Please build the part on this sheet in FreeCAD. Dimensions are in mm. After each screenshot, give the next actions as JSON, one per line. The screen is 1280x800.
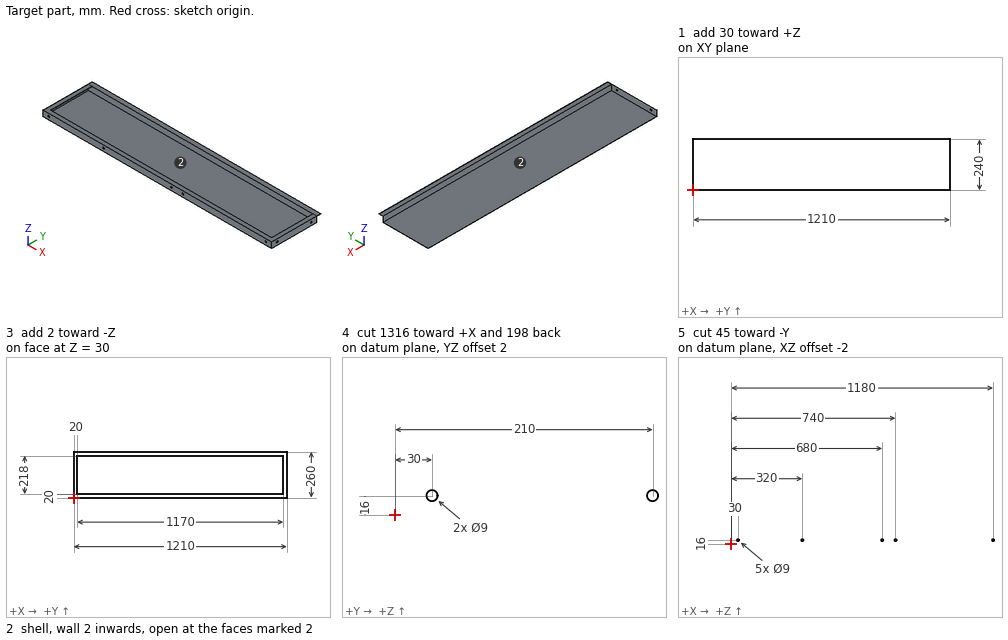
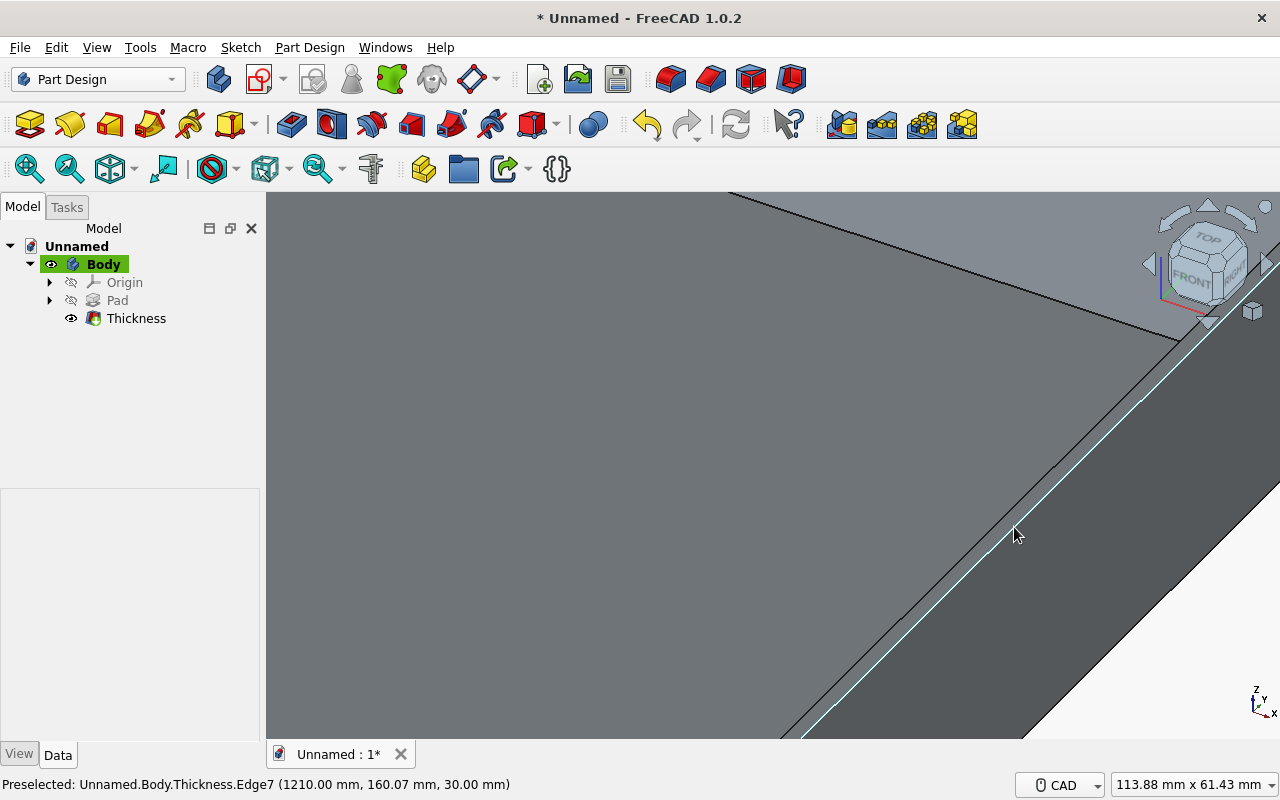
{"action": "scroll", "coordinate": [994, 539], "scroll_direction": "up", "scroll_amount": 4}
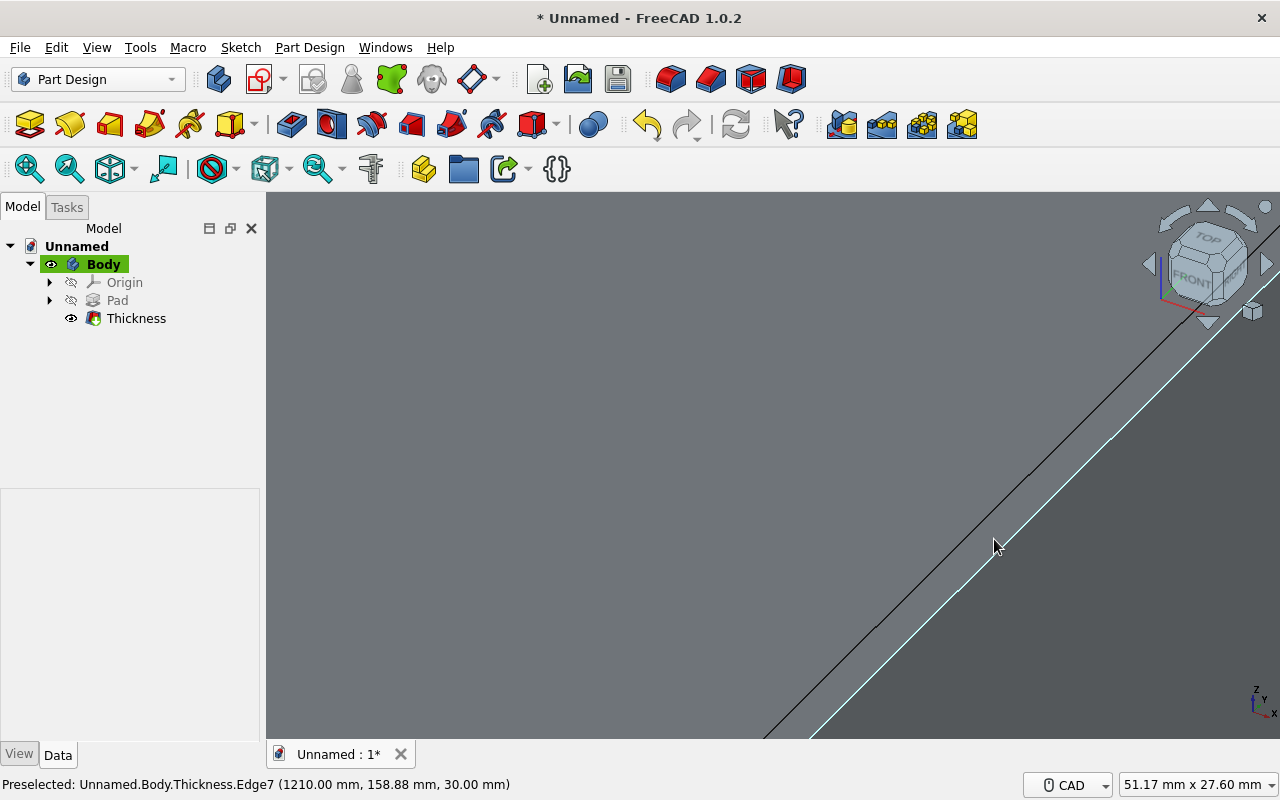
{"action": "left_click", "coordinate": [994, 539]}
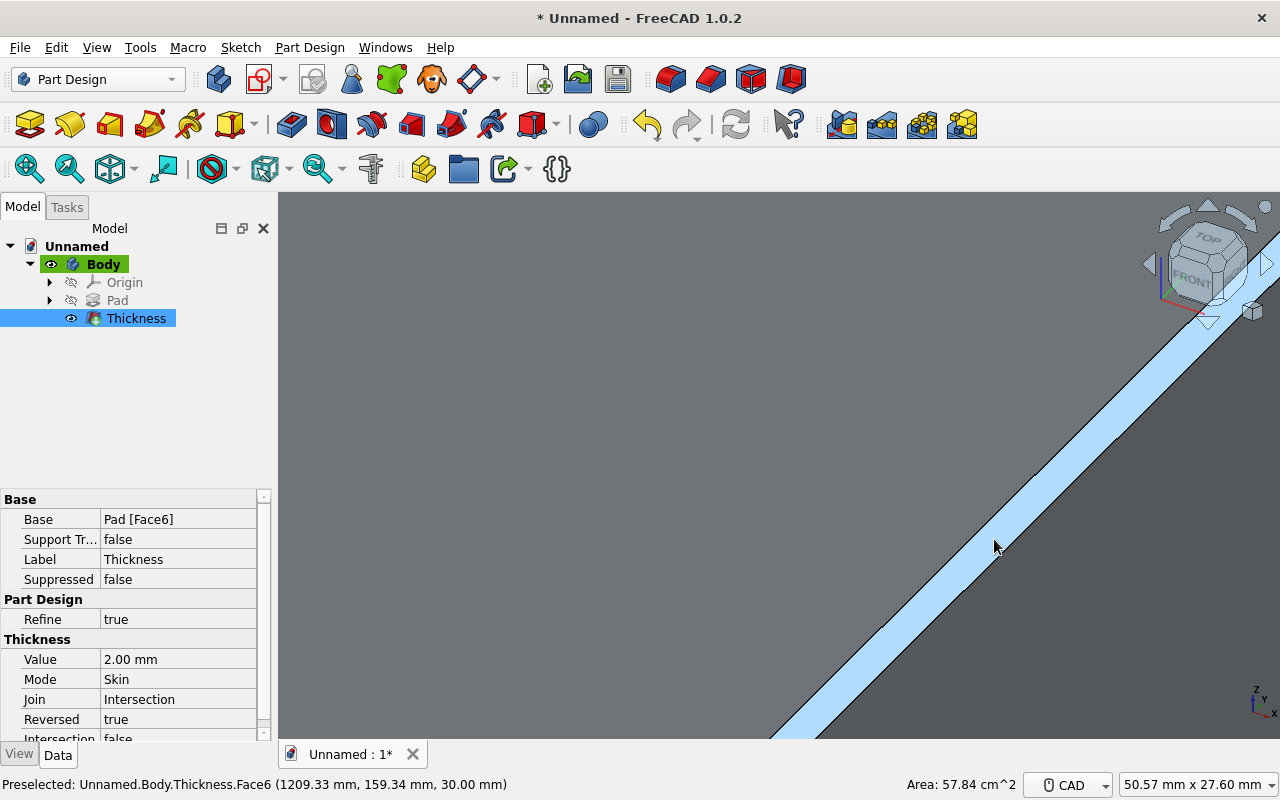
{"action": "left_click", "coordinate": [260, 80]}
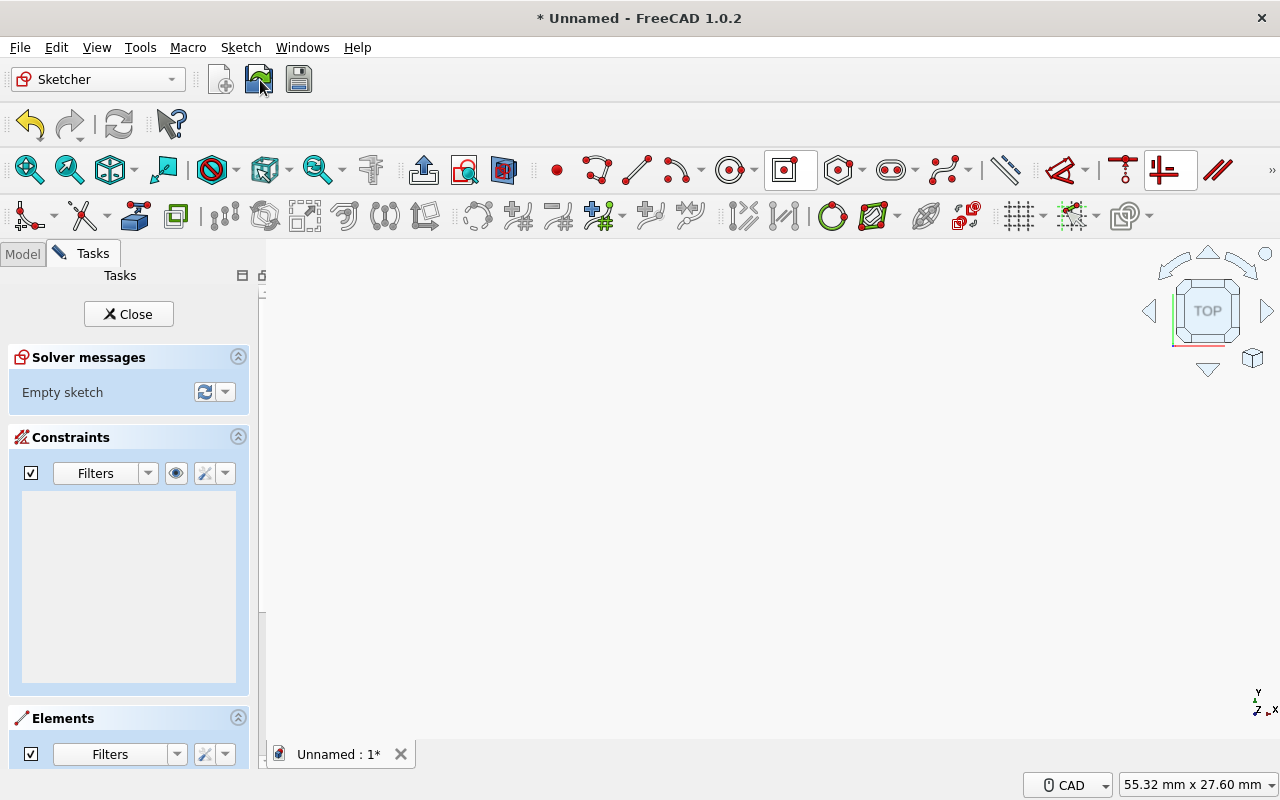
{"action": "scroll", "coordinate": [1015, 372], "scroll_direction": "down", "scroll_amount": 17}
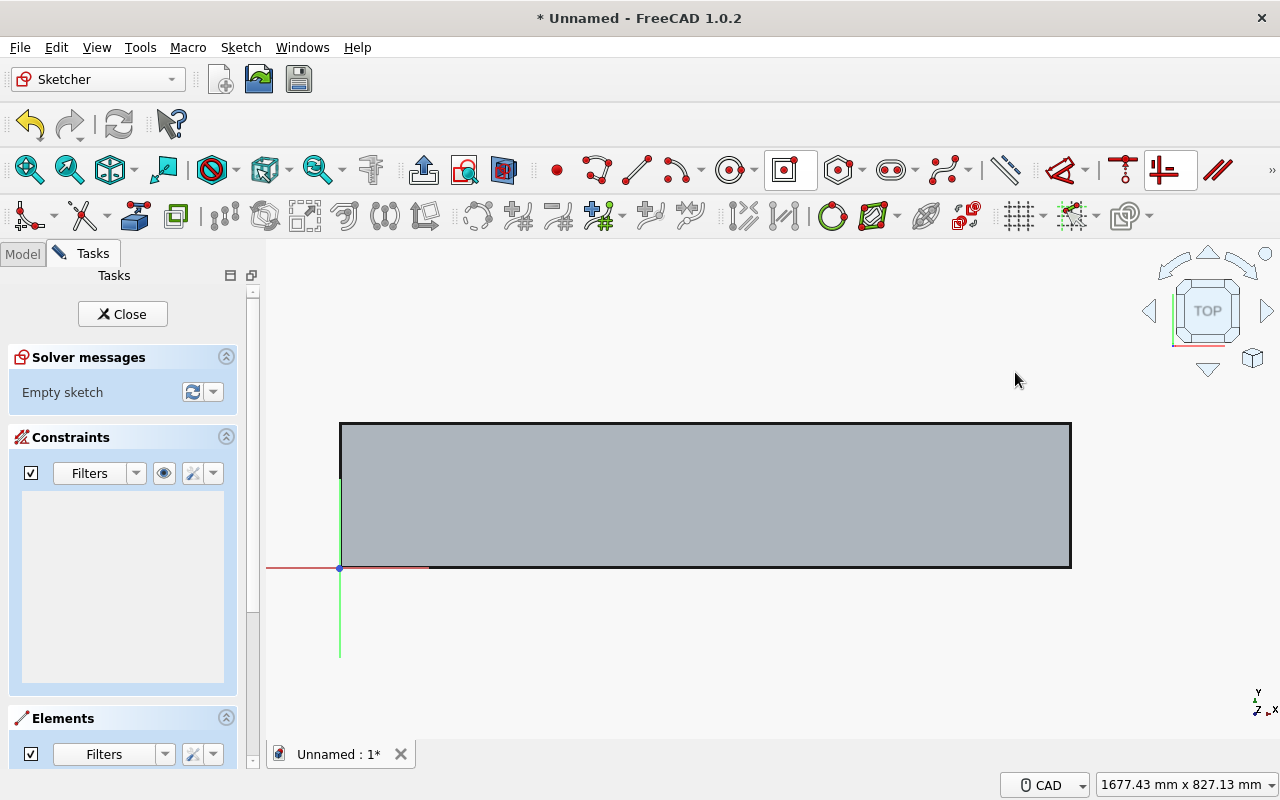
{"action": "left_click", "coordinate": [812, 170]}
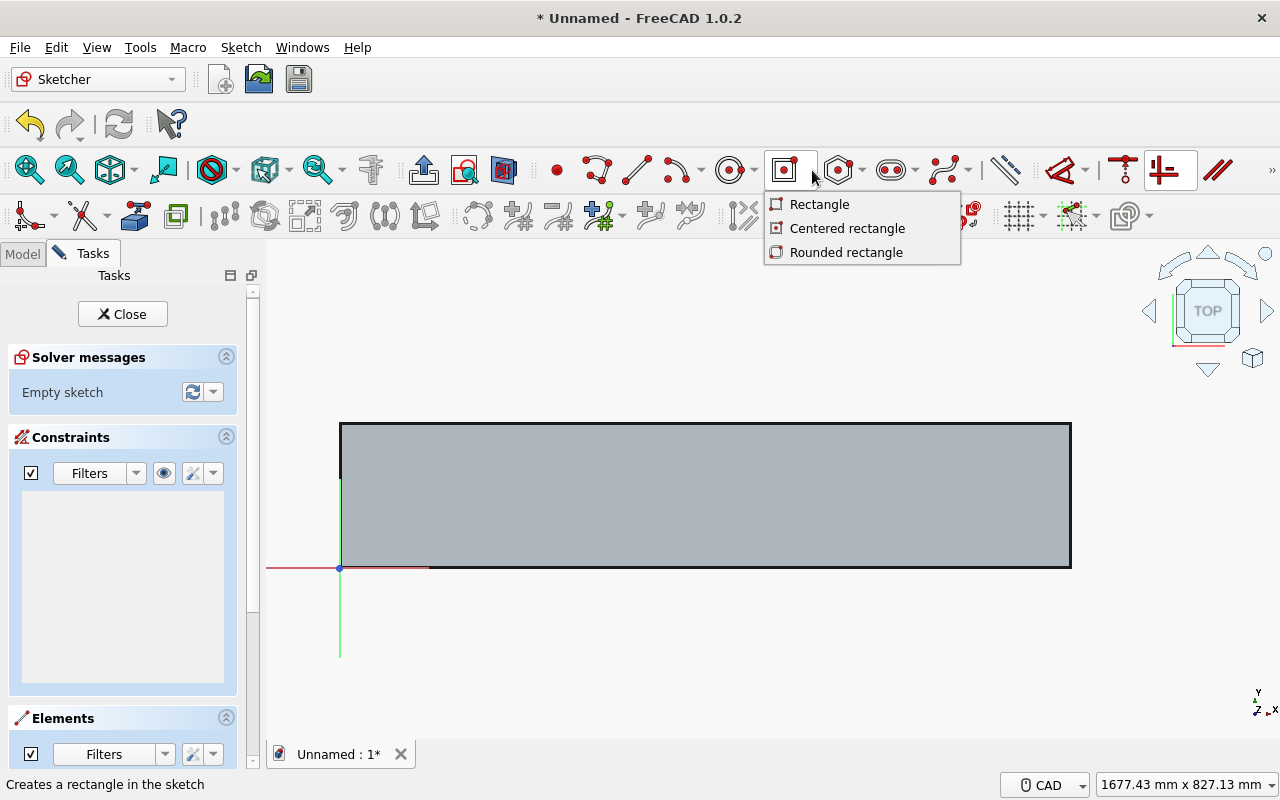
{"action": "left_click", "coordinate": [862, 204]}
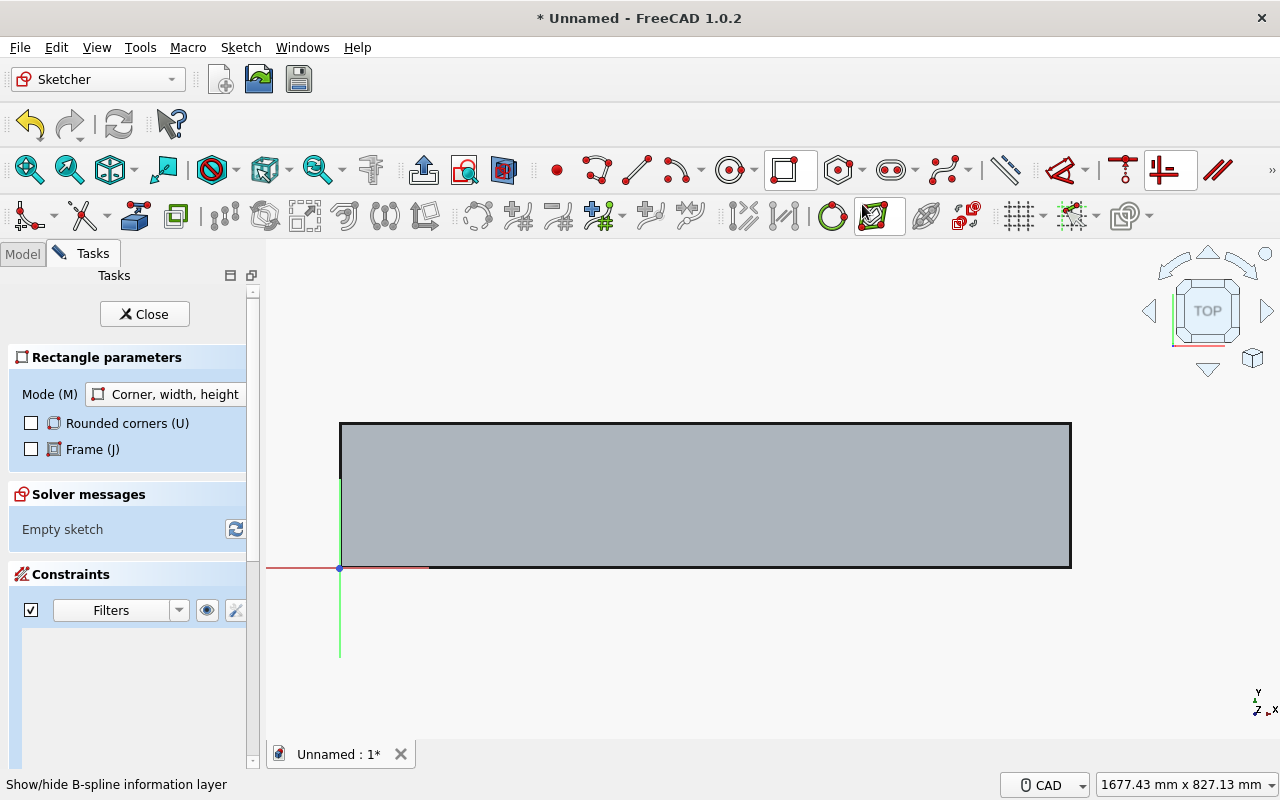
{"action": "left_click", "coordinate": [340, 568]}
{"action": "mouse_move", "coordinate": [1071, 411]}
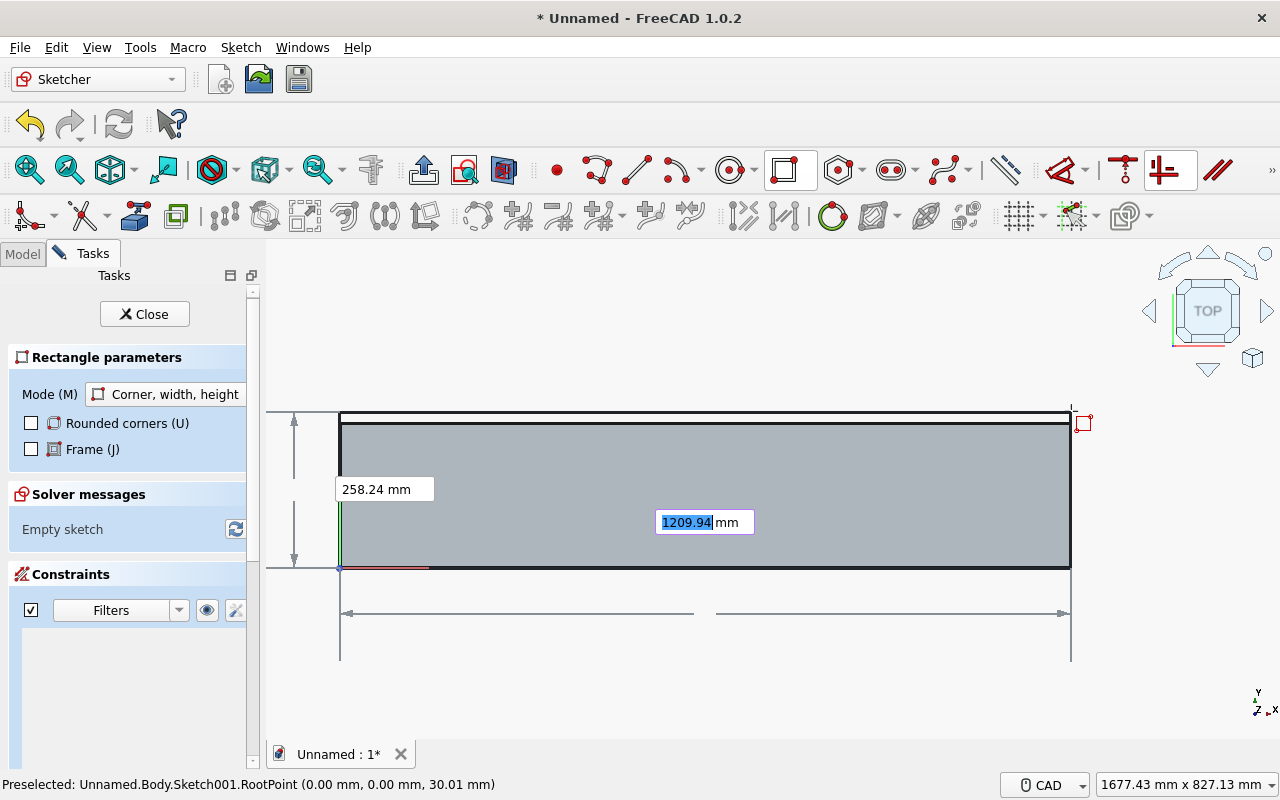
{"action": "type", "text": "1210"}
{"action": "key", "text": "Tab"}
{"action": "type", "text": "260"}
{"action": "key", "text": "Return"}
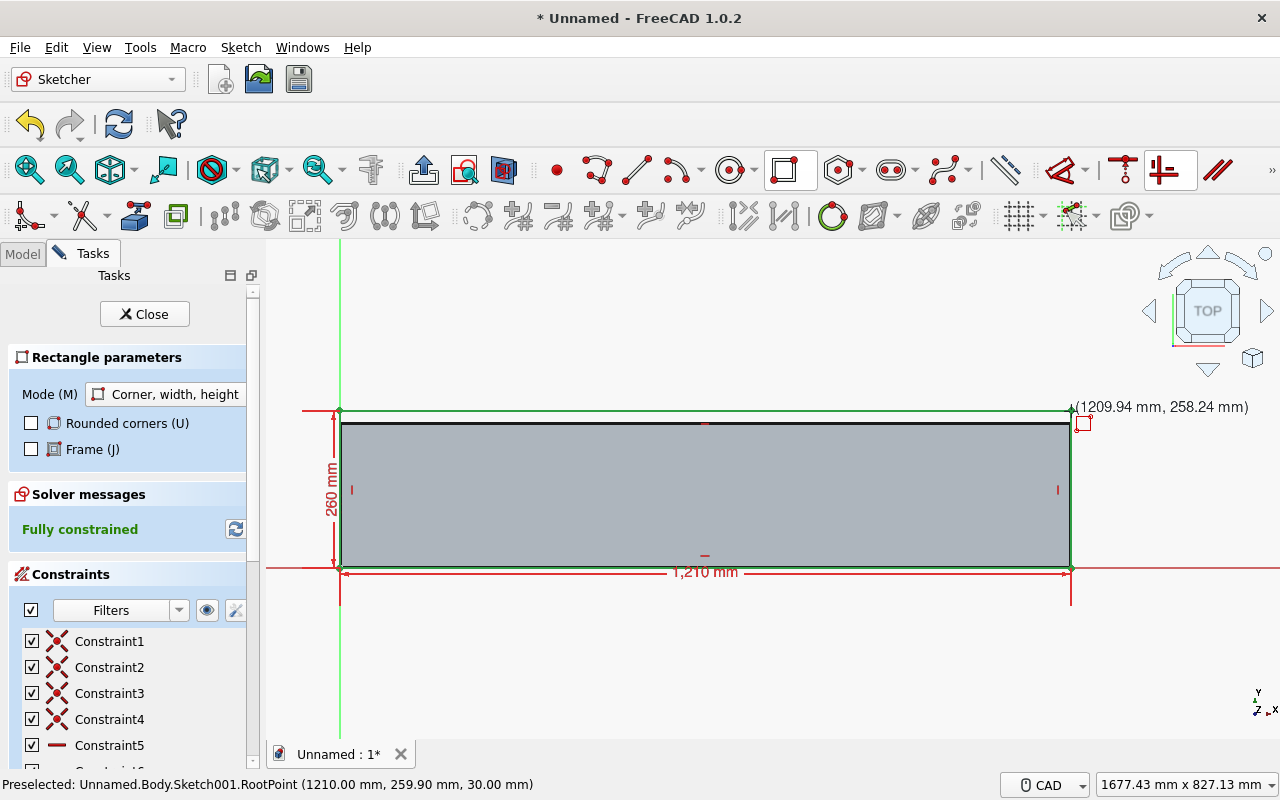
{"action": "scroll", "coordinate": [352, 424], "scroll_direction": "up", "scroll_amount": 2}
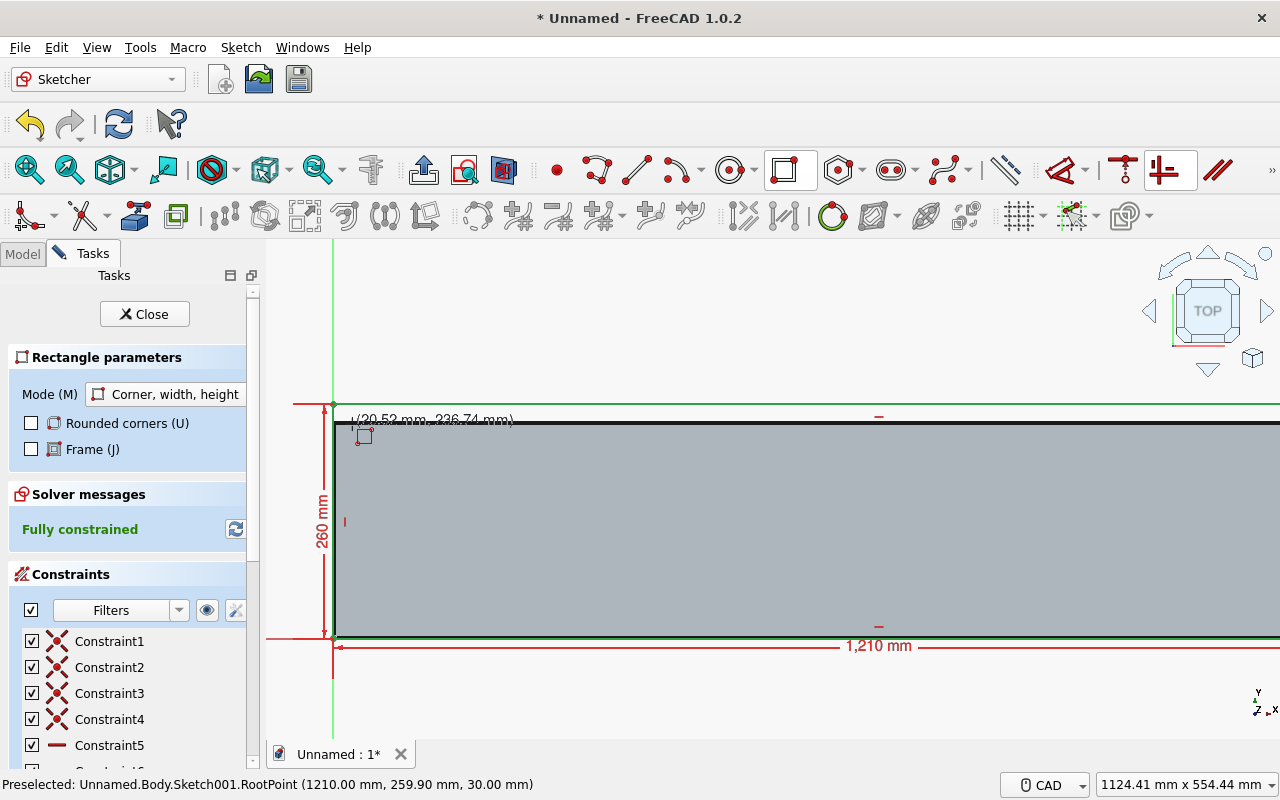
{"action": "left_click", "coordinate": [351, 424]}